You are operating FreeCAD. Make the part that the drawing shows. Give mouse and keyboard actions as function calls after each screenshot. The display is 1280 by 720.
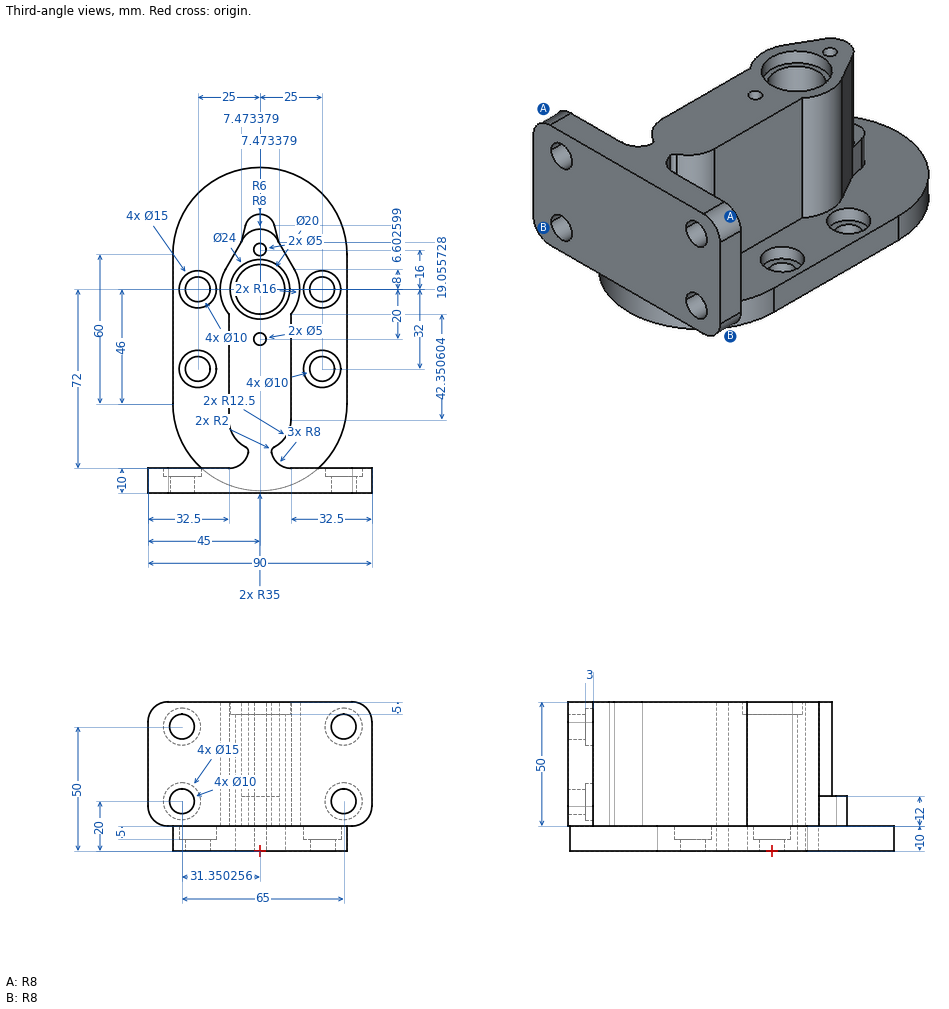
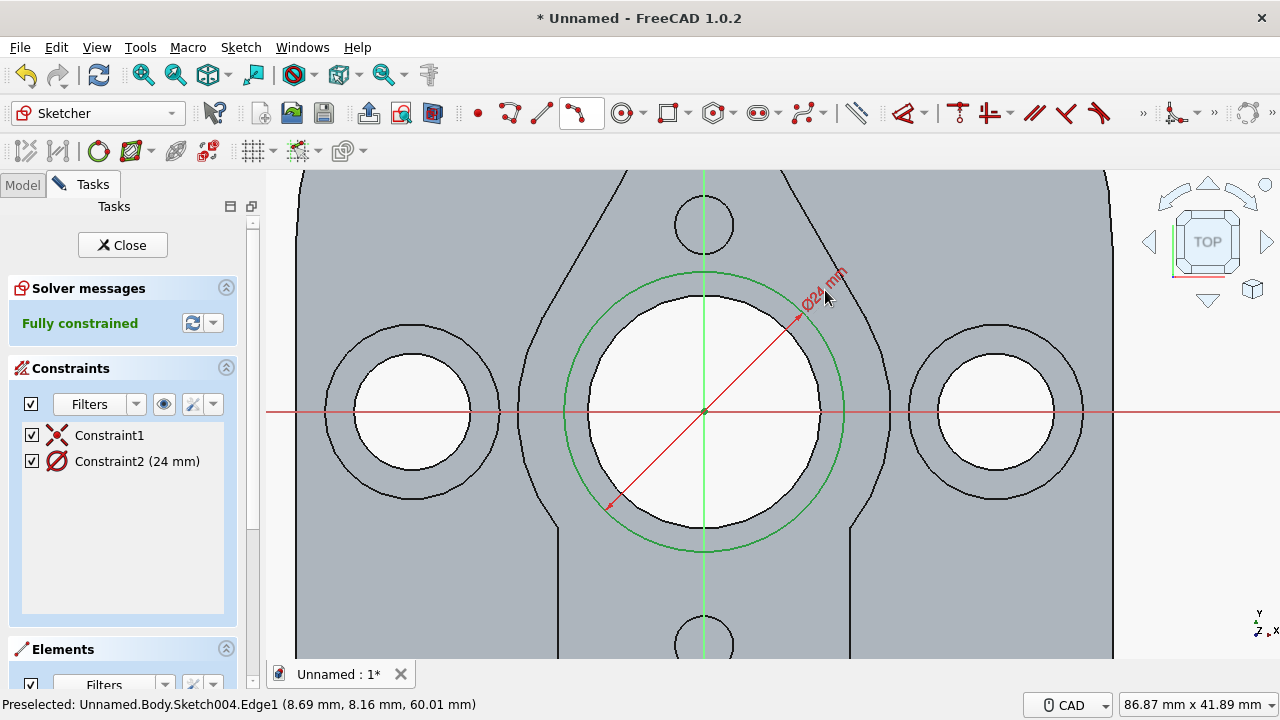
click(123, 245)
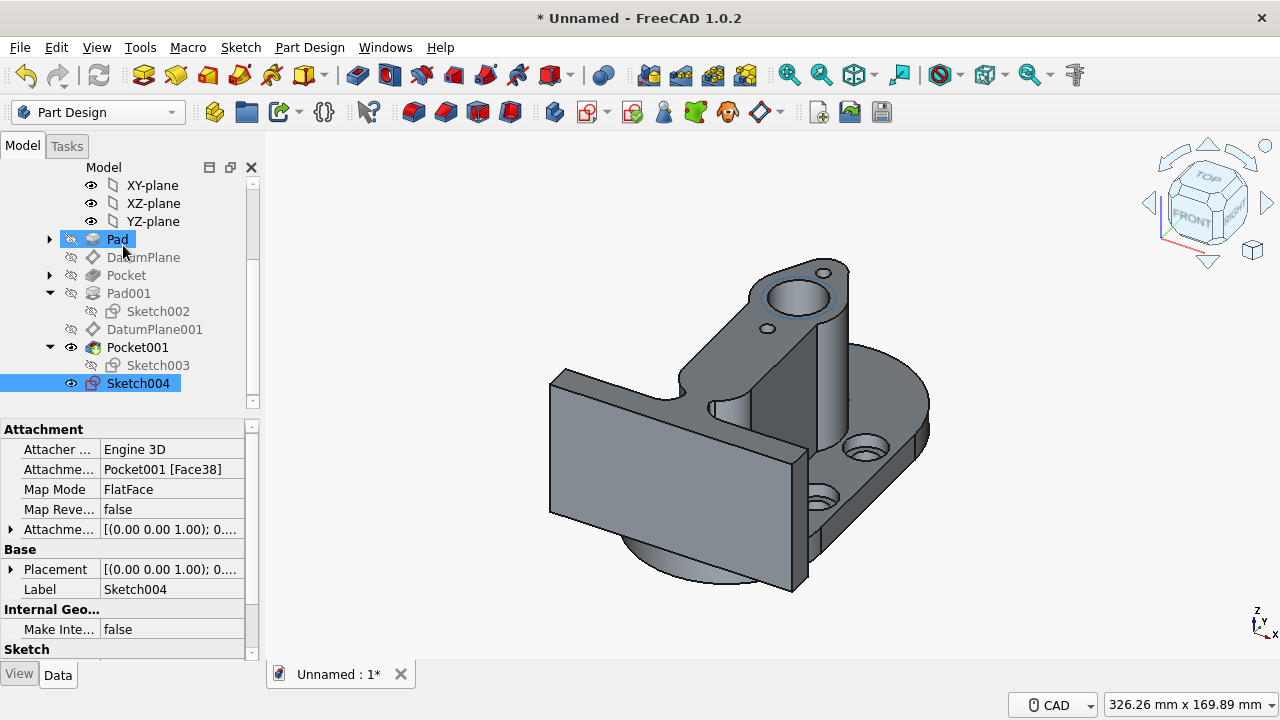
click(358, 76)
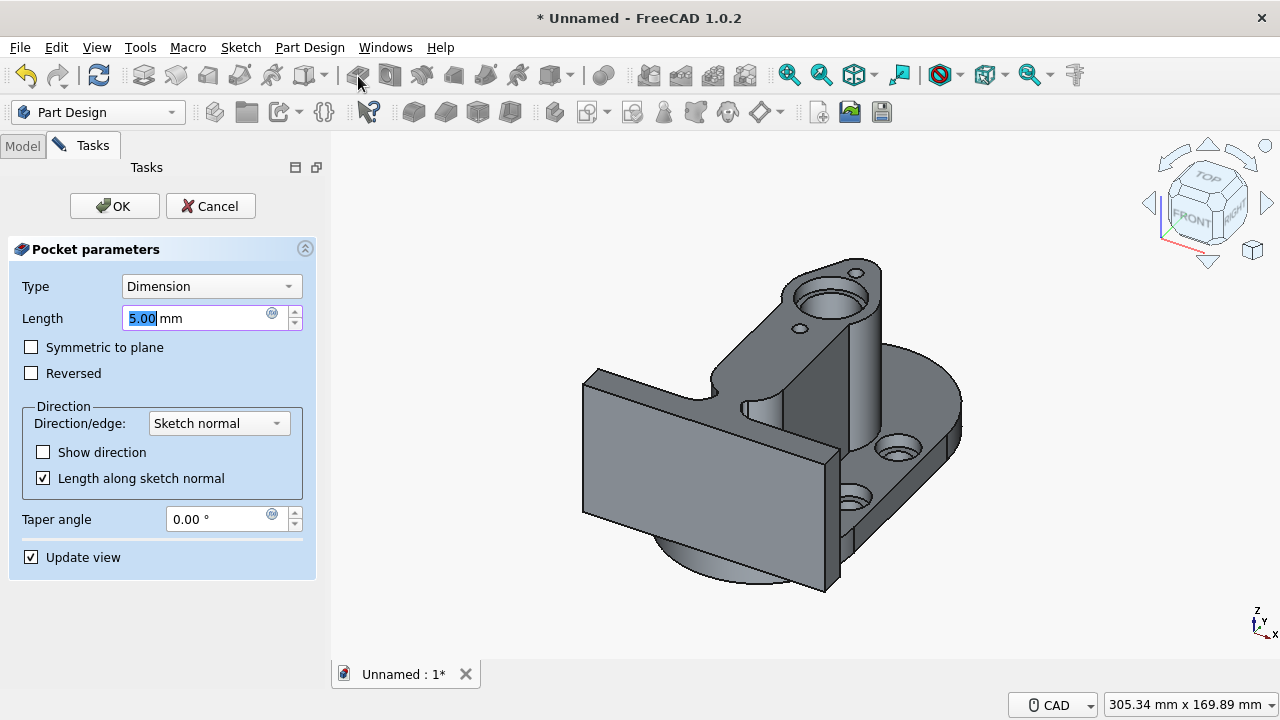
text(5)
key(Tab)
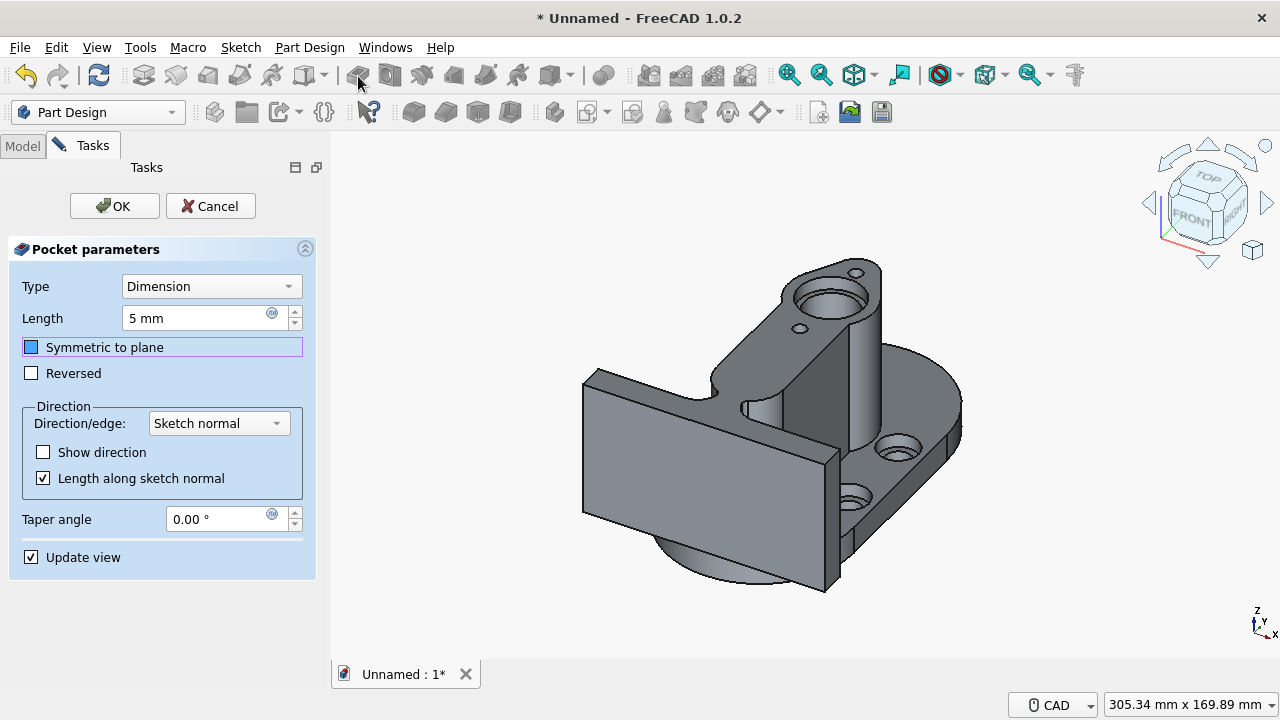
click(115, 206)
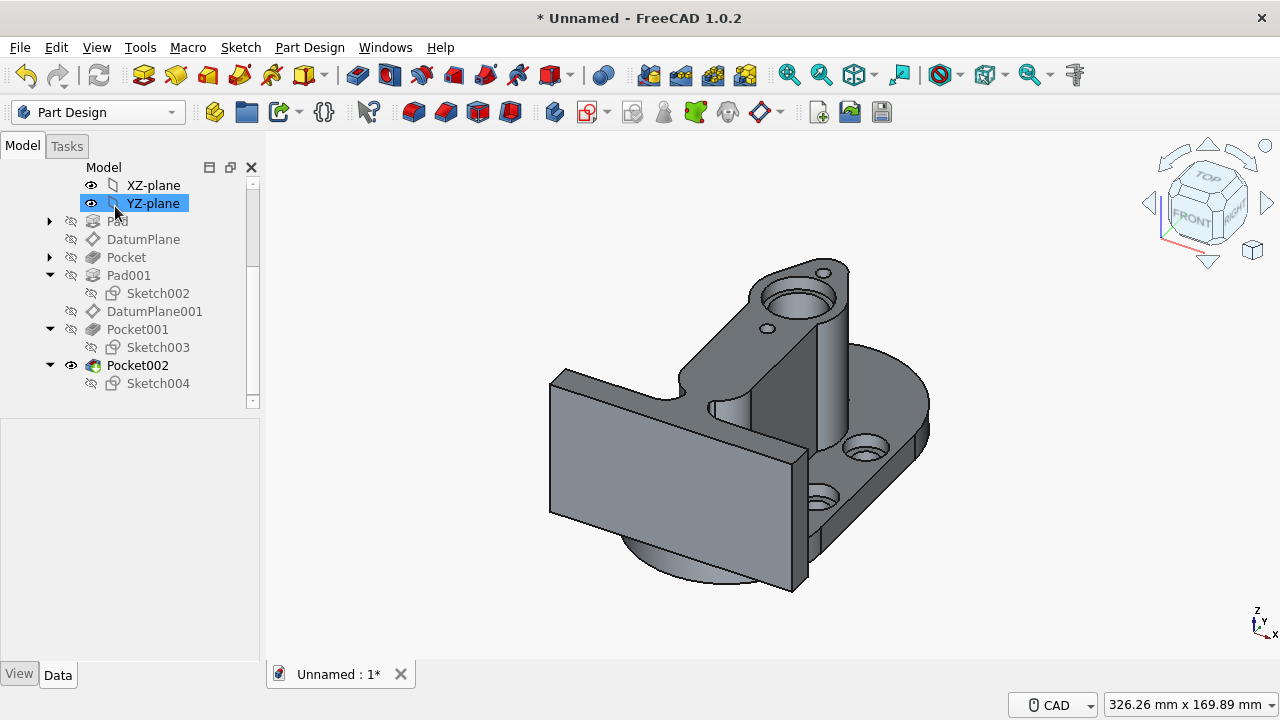
key(4)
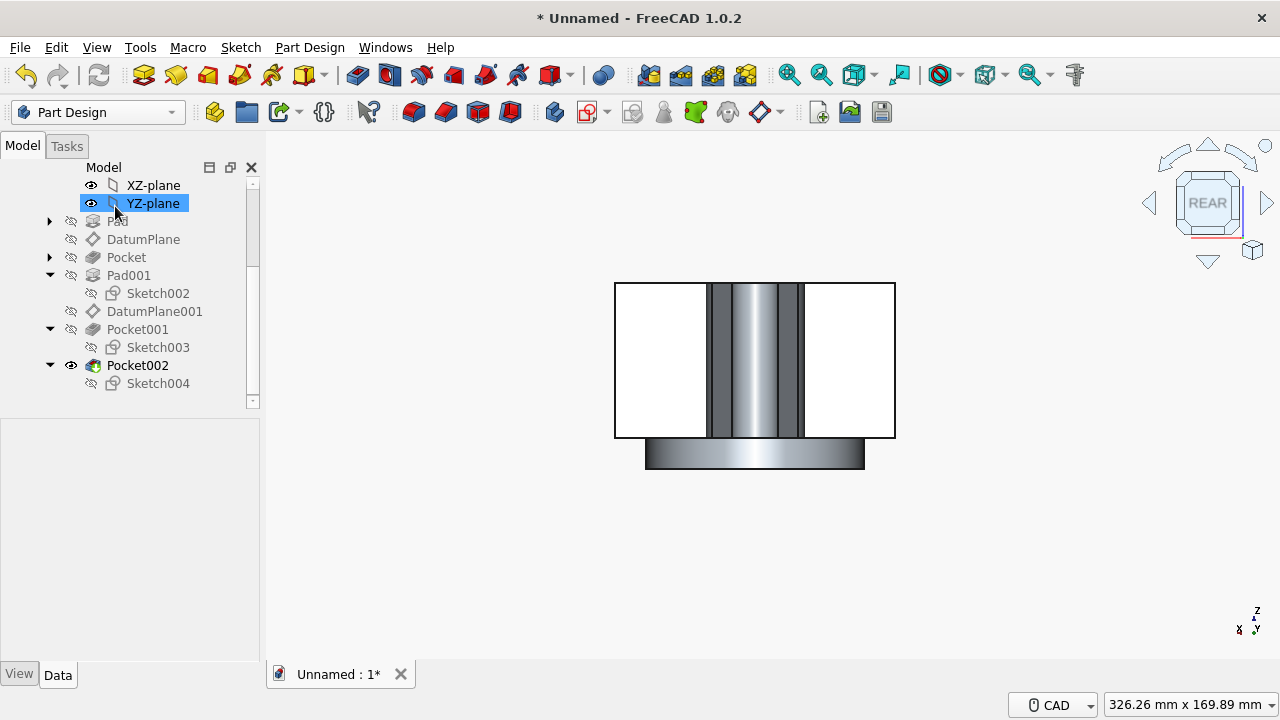
click(790, 76)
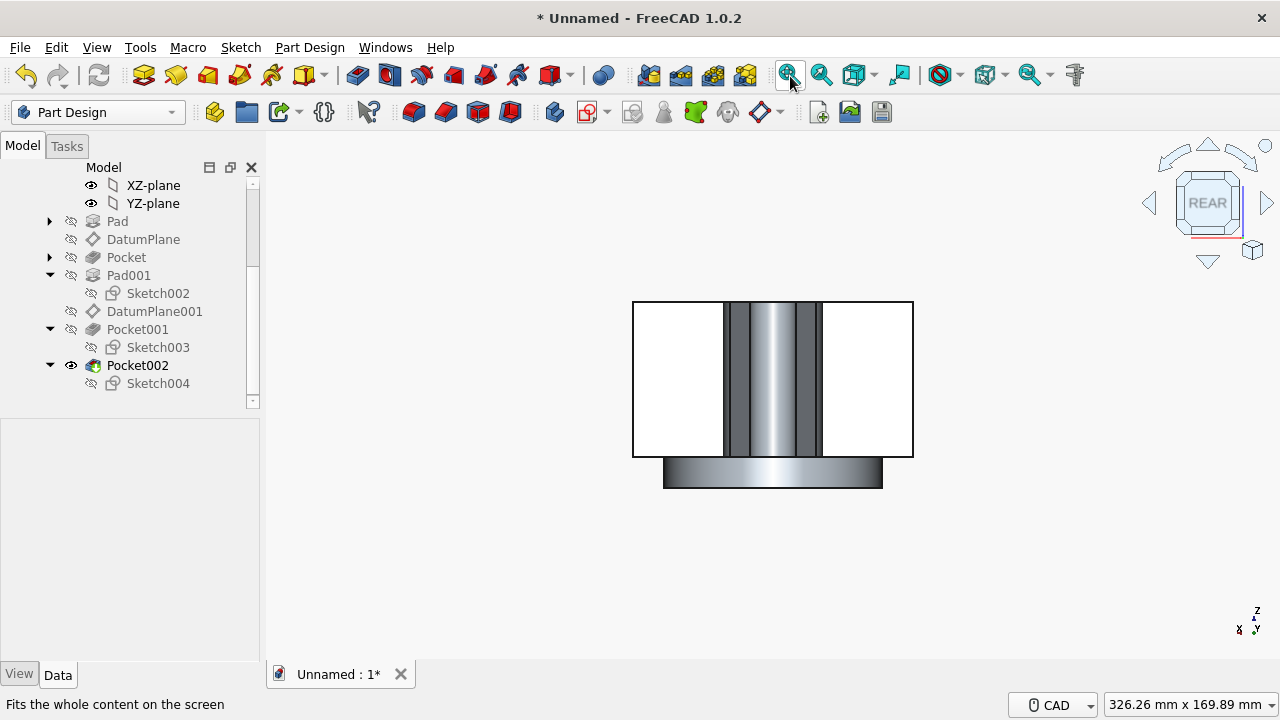
click(862, 356)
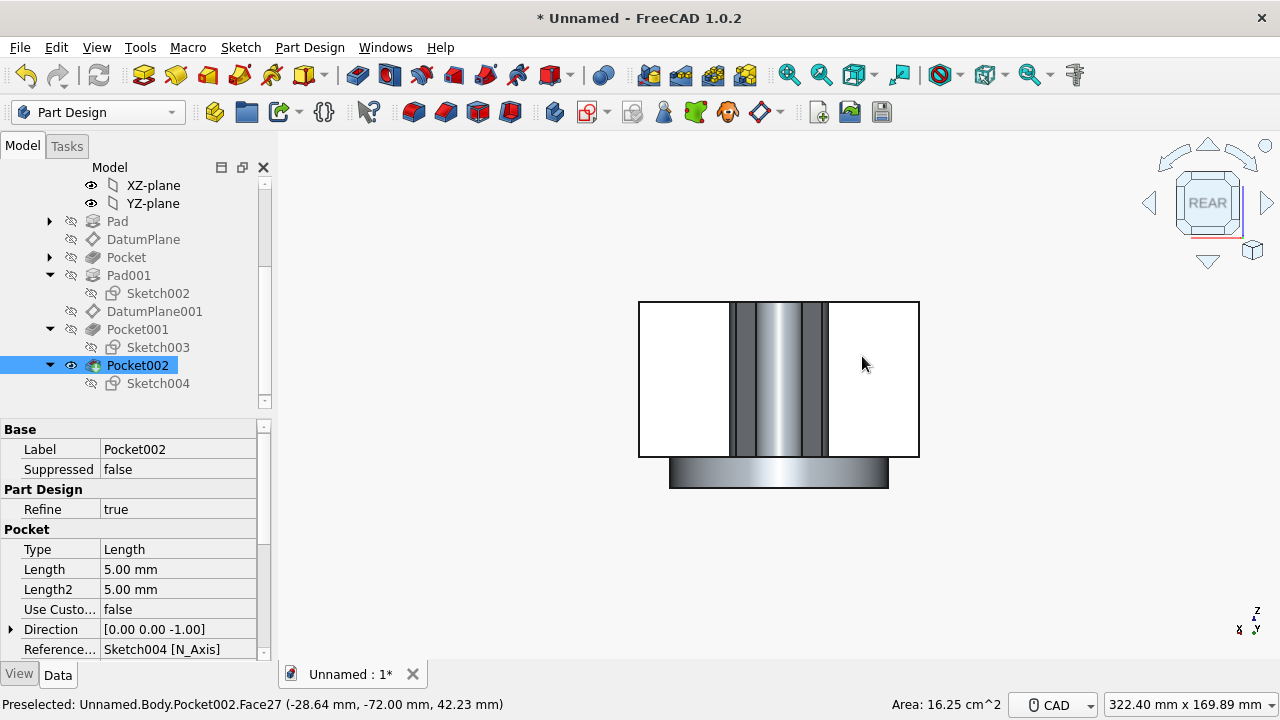
click(588, 112)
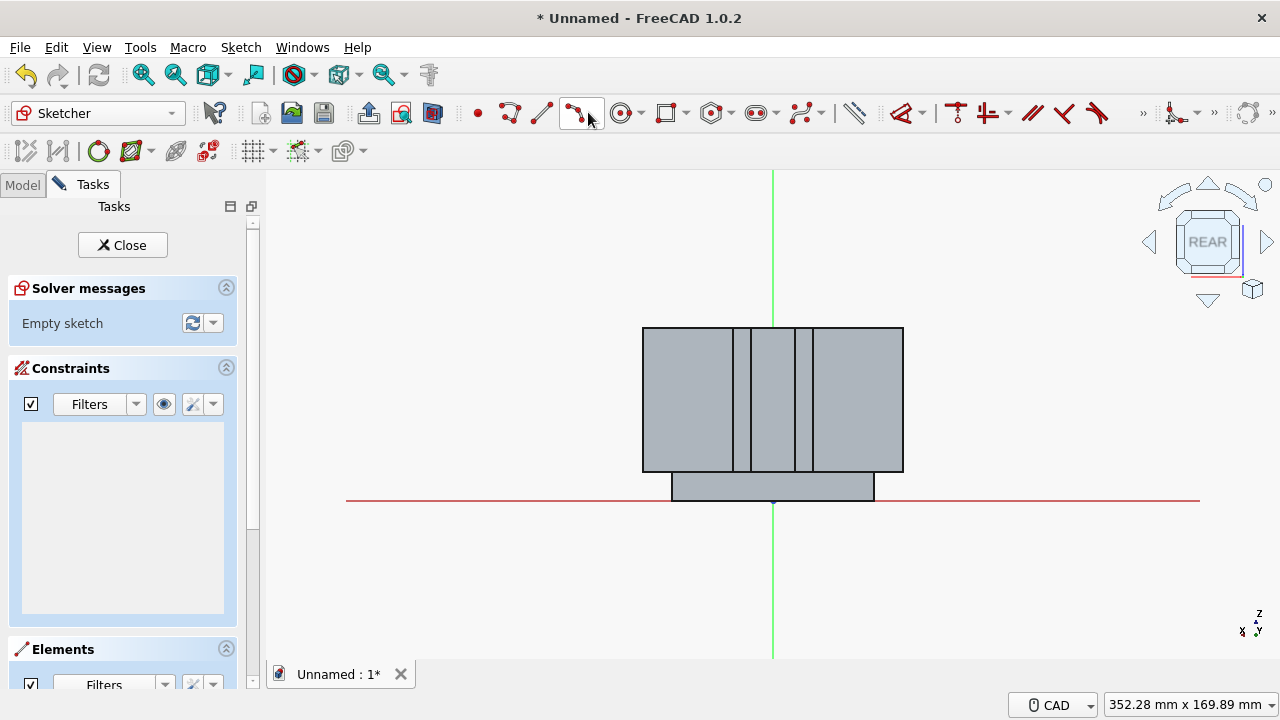
click(434, 114)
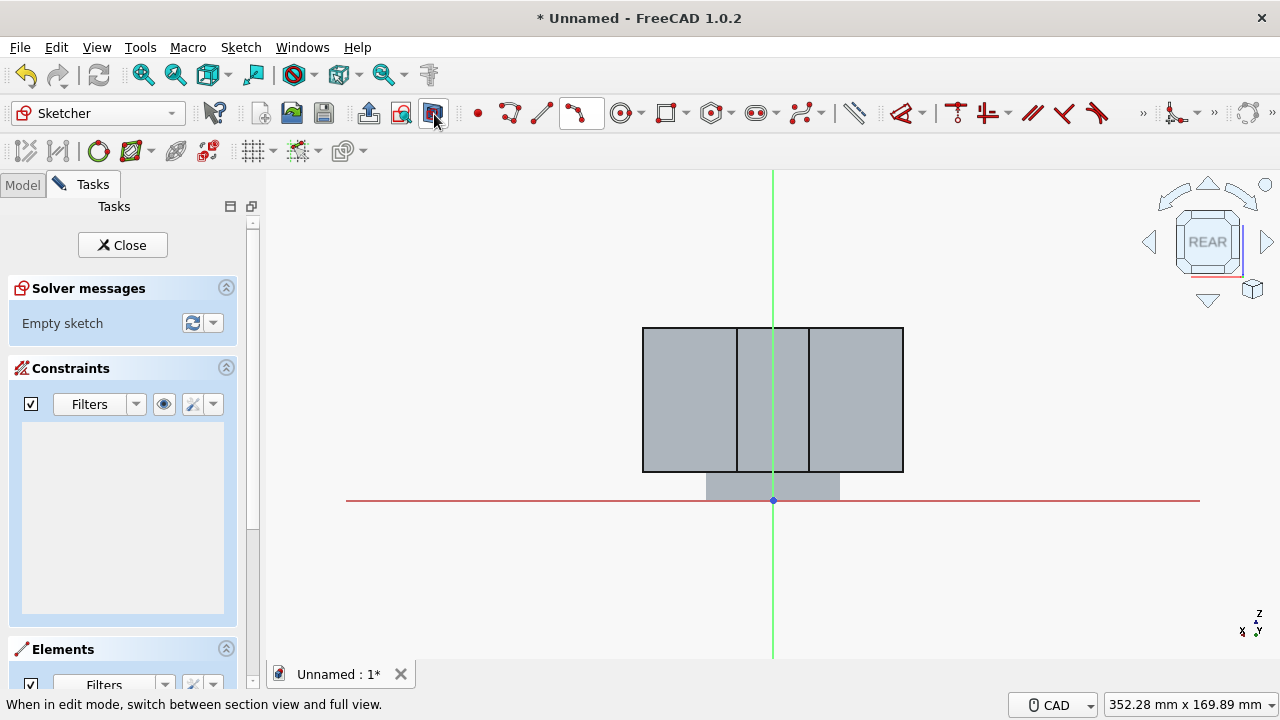
scroll(849, 430, up, 3)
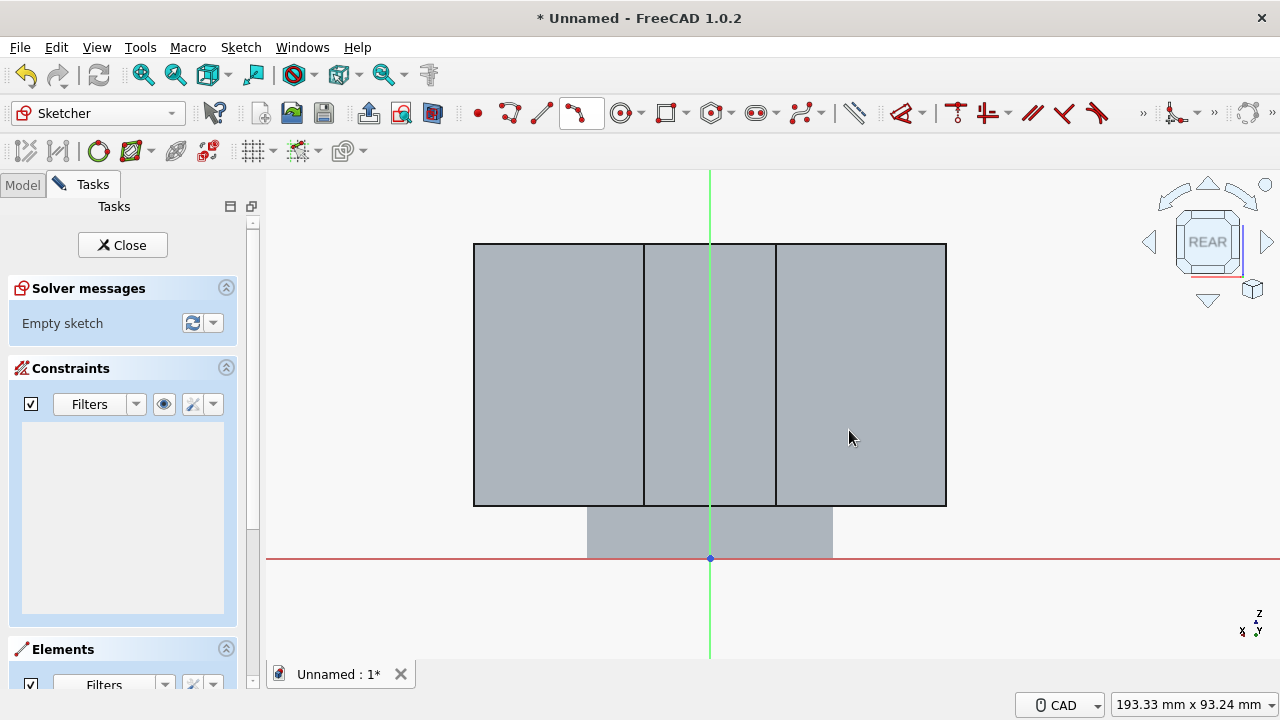
click(622, 114)